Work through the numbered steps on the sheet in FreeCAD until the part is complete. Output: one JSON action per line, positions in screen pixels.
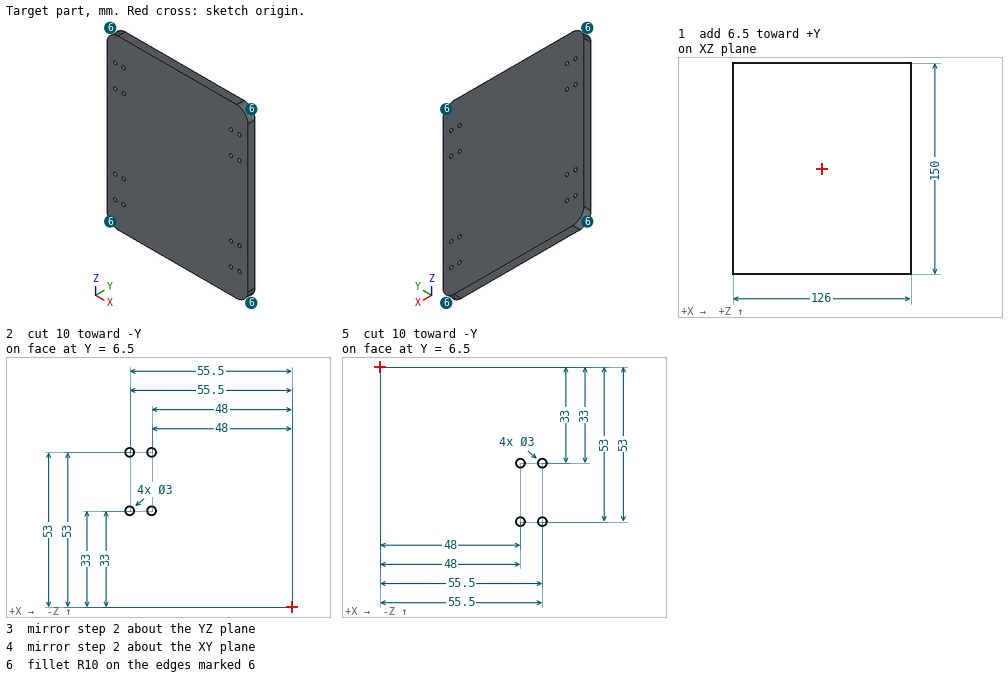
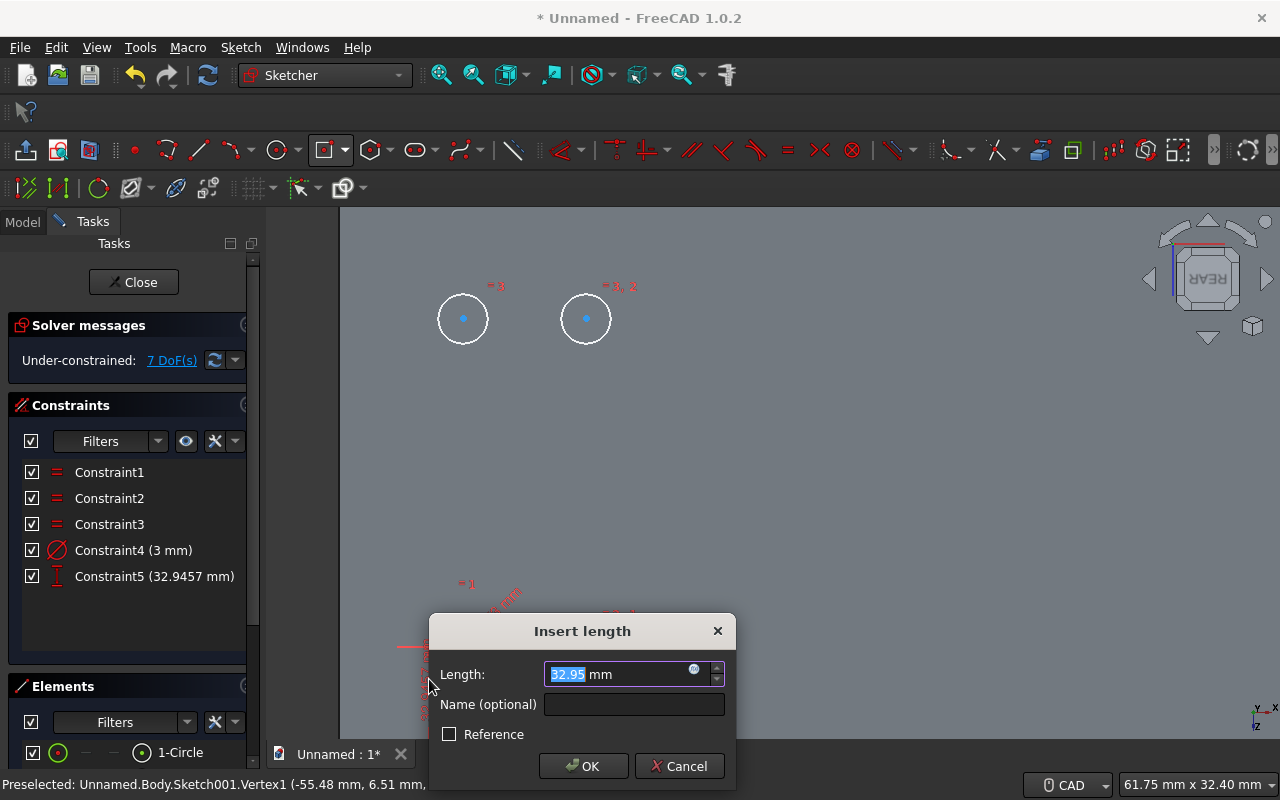
{"action": "type", "text": "33"}
{"action": "key", "text": "Return"}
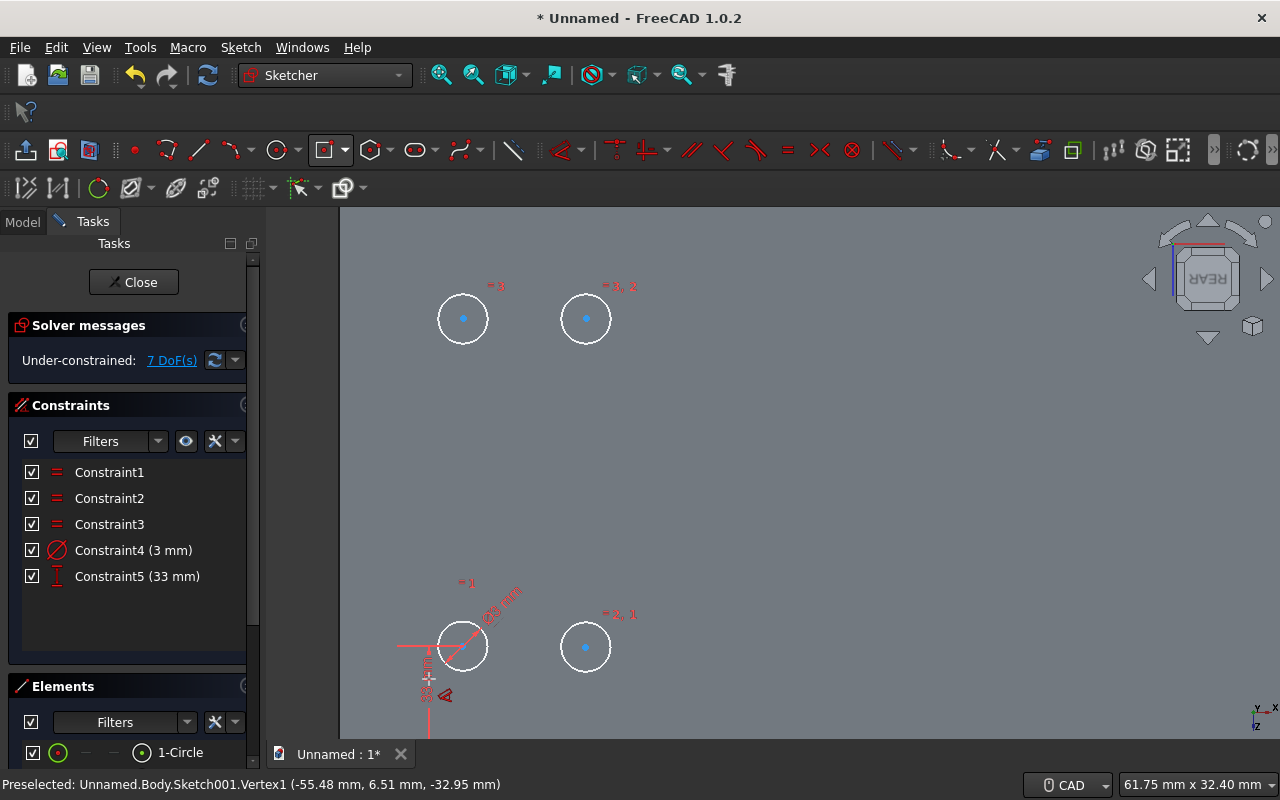
{"action": "left_click", "coordinate": [586, 647]}
{"action": "left_click", "coordinate": [850, 613]}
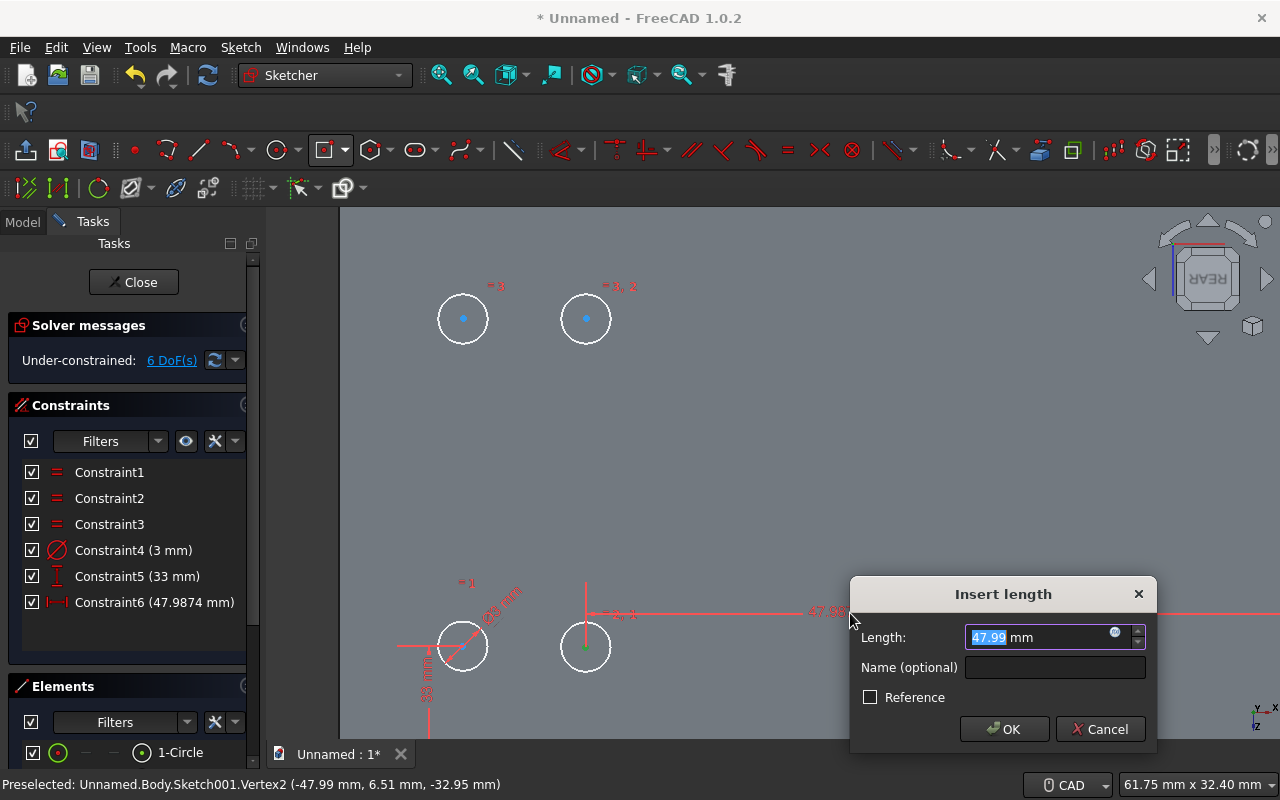
{"action": "type", "text": "48"}
{"action": "key", "text": "Return"}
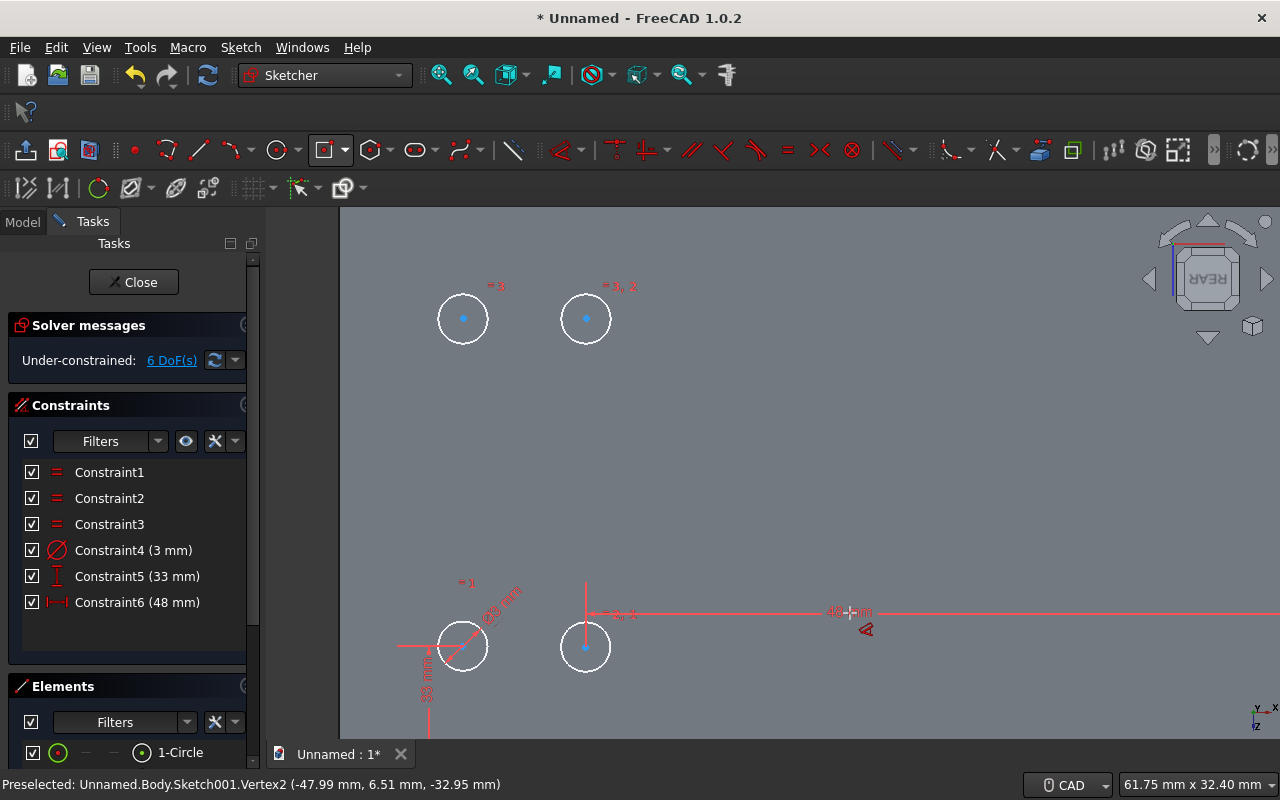
{"action": "left_click", "coordinate": [586, 647]}
{"action": "left_click", "coordinate": [552, 679]}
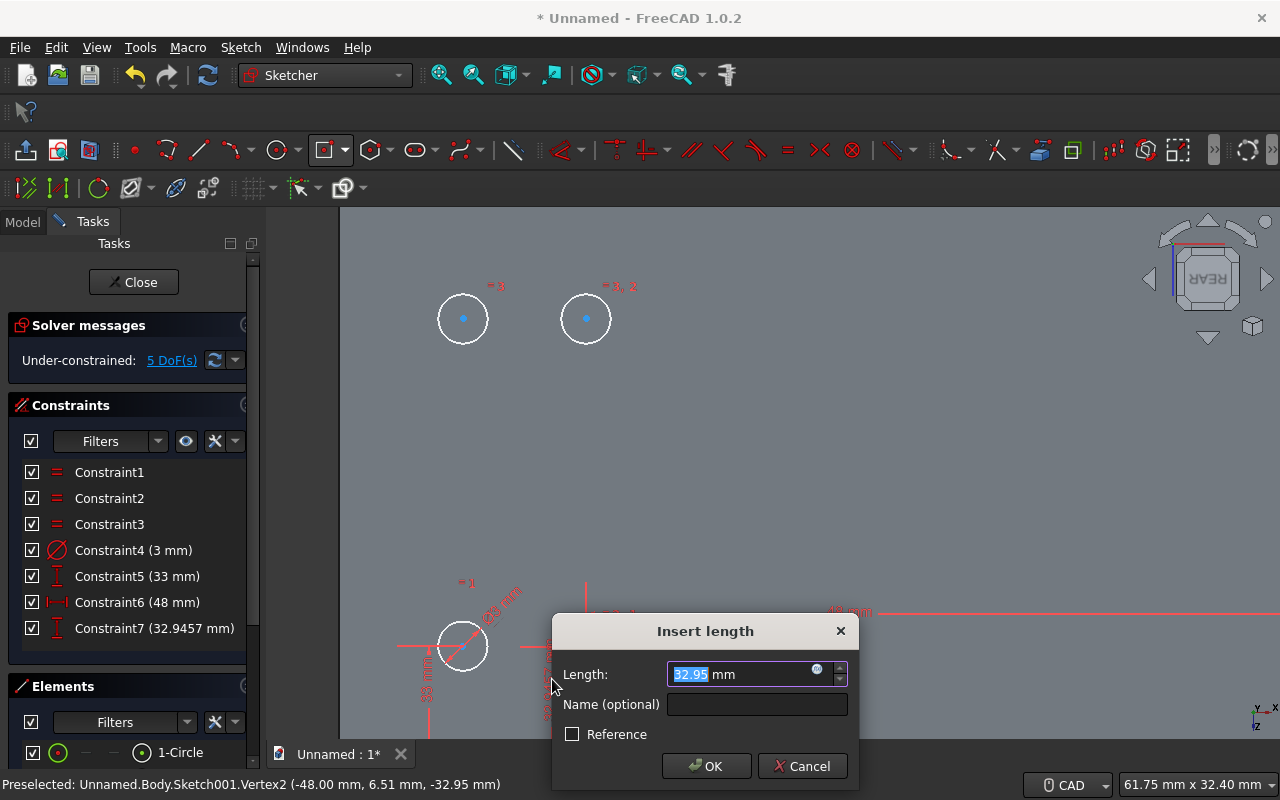
{"action": "type", "text": "33"}
{"action": "key", "text": "Return"}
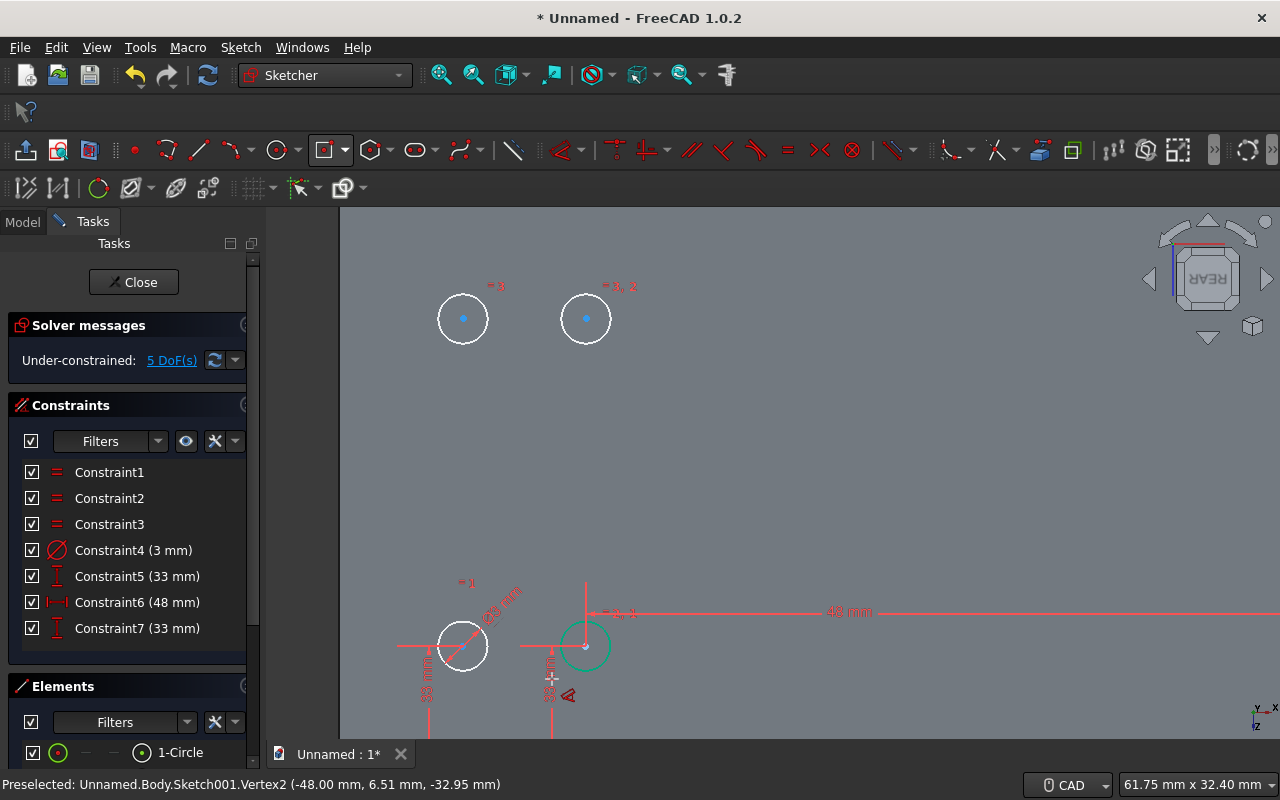
{"action": "left_click", "coordinate": [586, 319]}
{"action": "left_click", "coordinate": [850, 285]}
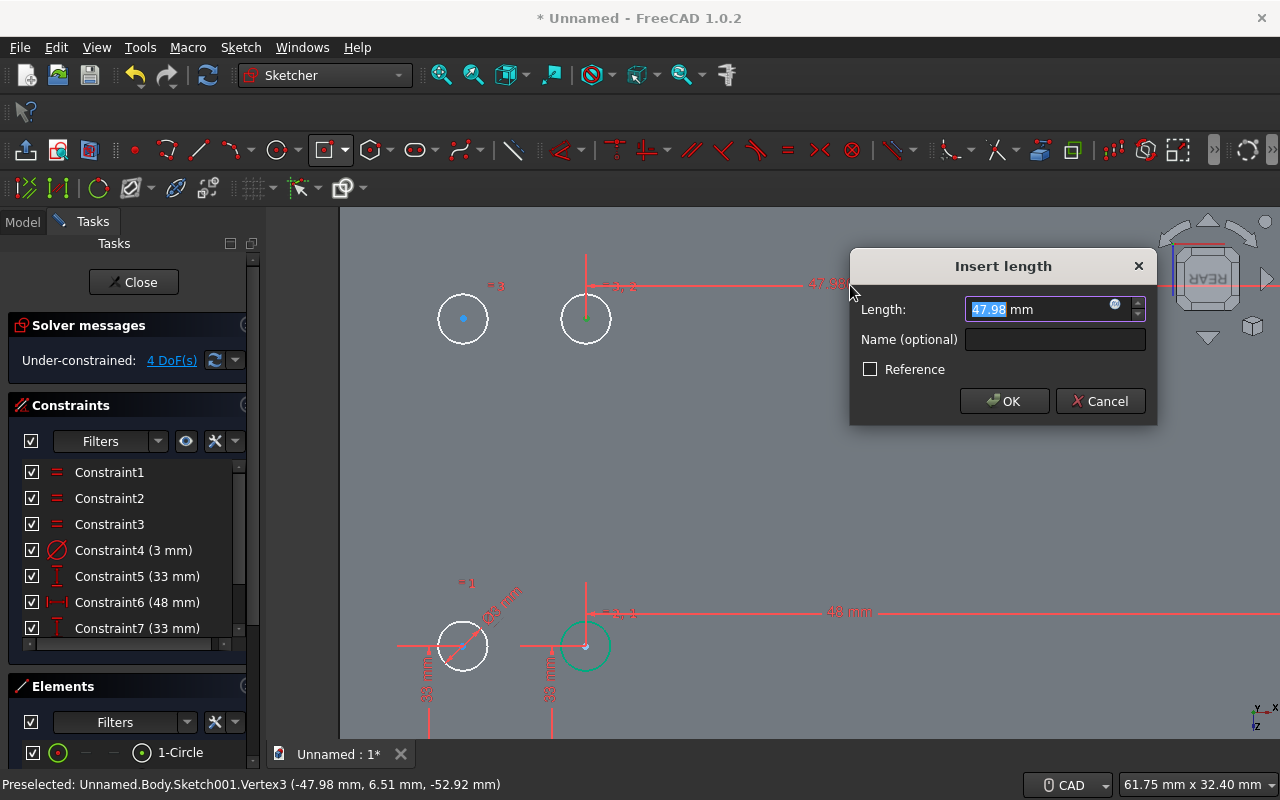
{"action": "type", "text": "48"}
{"action": "key", "text": "Return"}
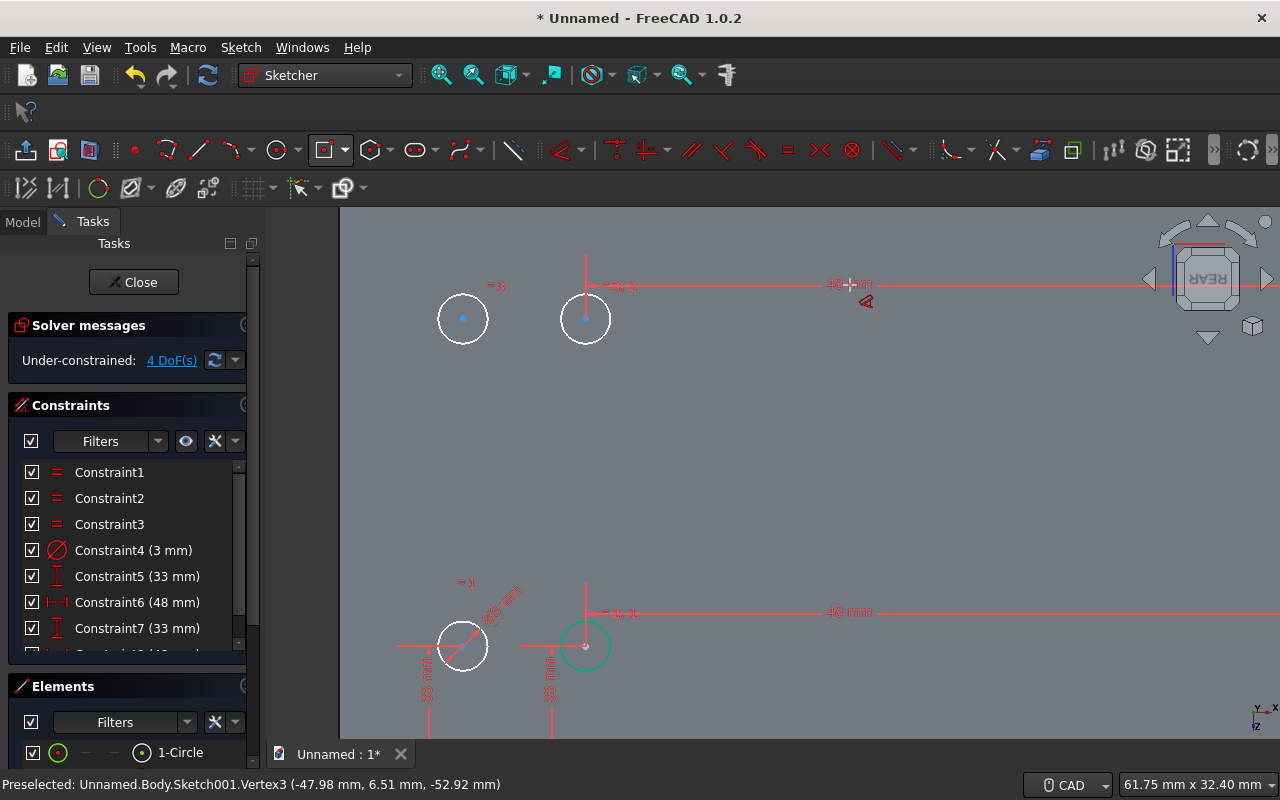
{"action": "left_click", "coordinate": [586, 319]}
{"action": "left_click", "coordinate": [552, 515]}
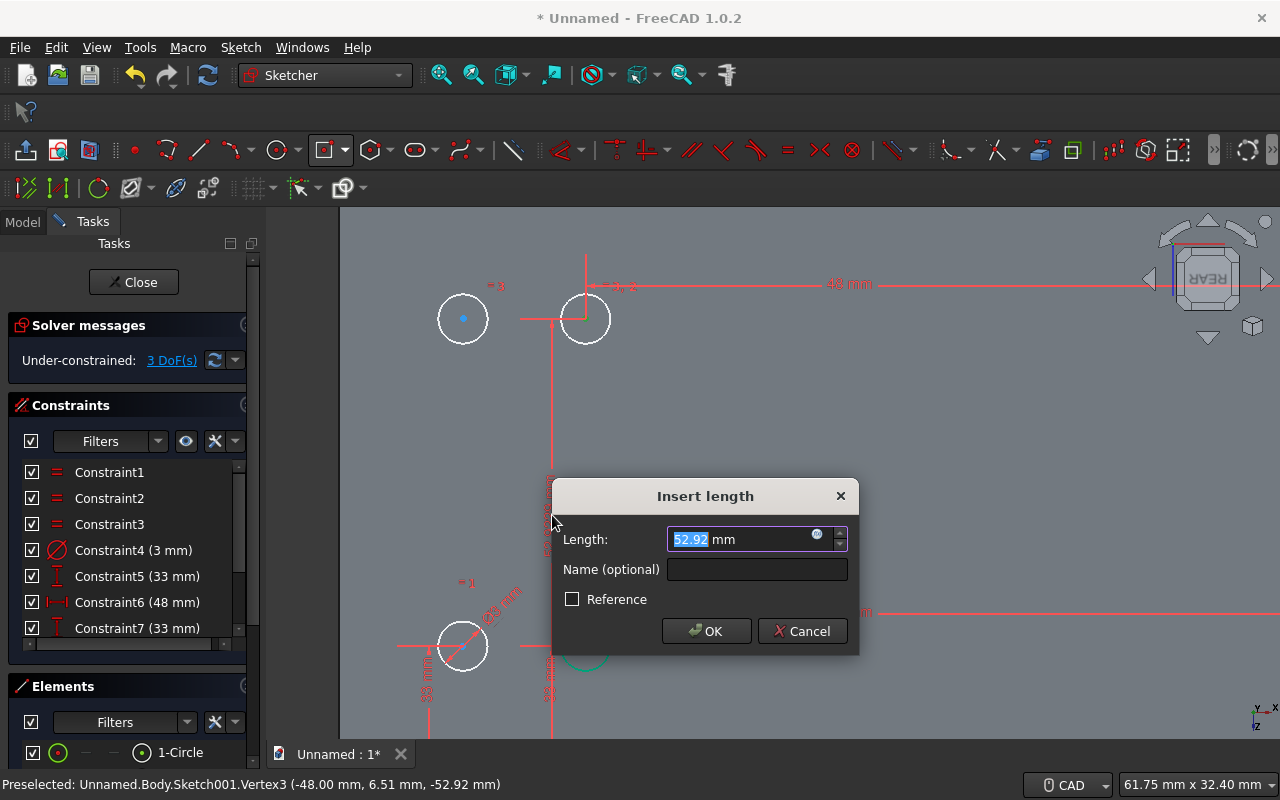
{"action": "type", "text": "53"}
{"action": "key", "text": "Return"}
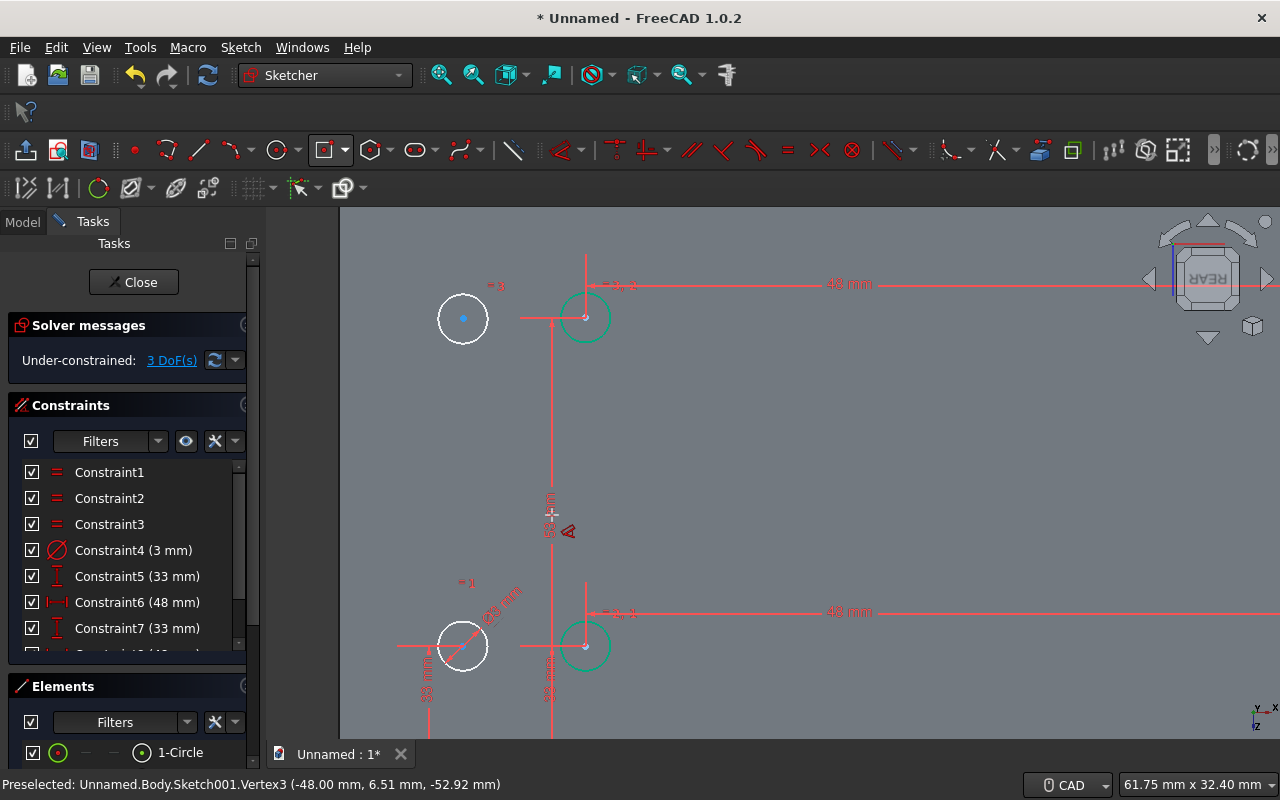
{"action": "left_click", "coordinate": [463, 319]}
{"action": "left_click", "coordinate": [429, 515]}